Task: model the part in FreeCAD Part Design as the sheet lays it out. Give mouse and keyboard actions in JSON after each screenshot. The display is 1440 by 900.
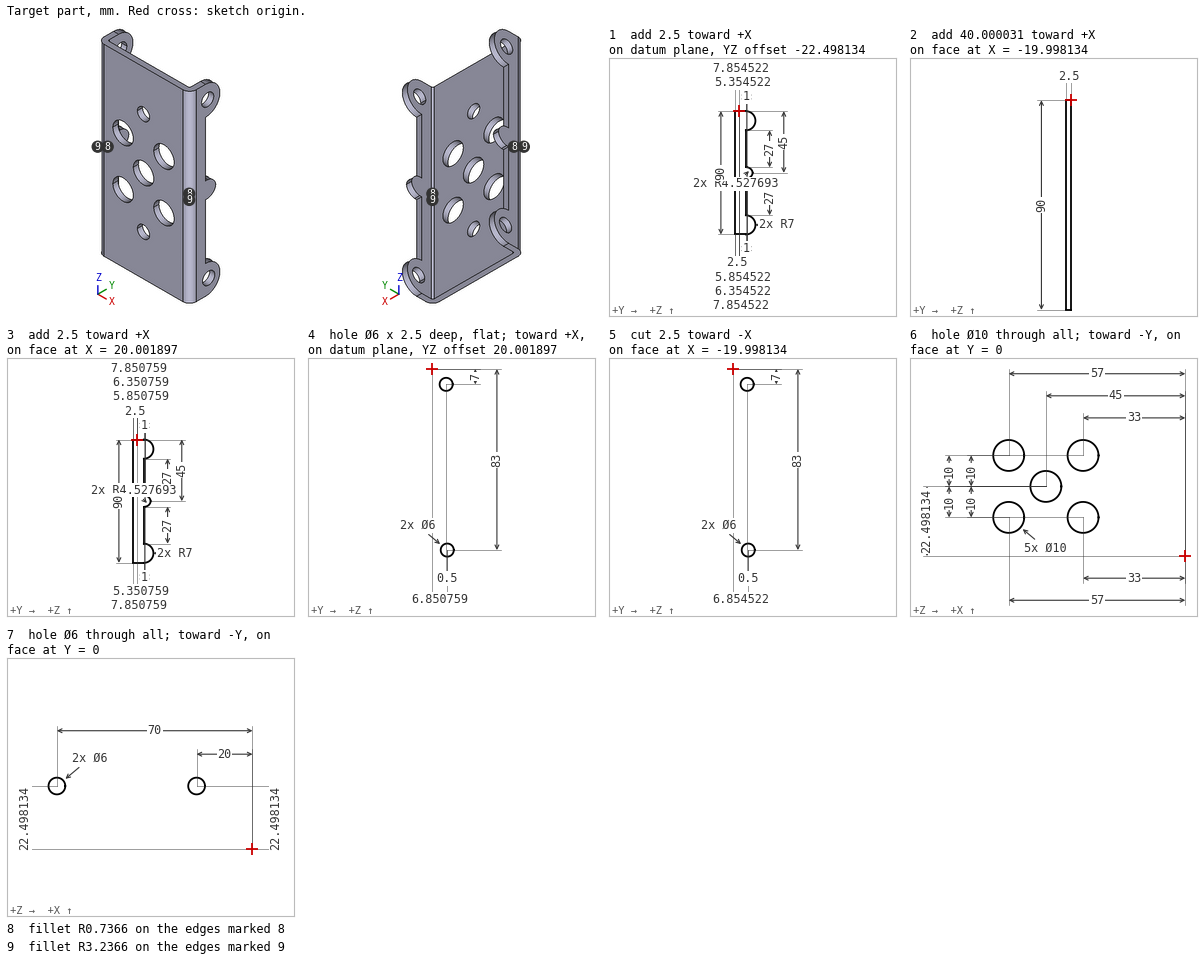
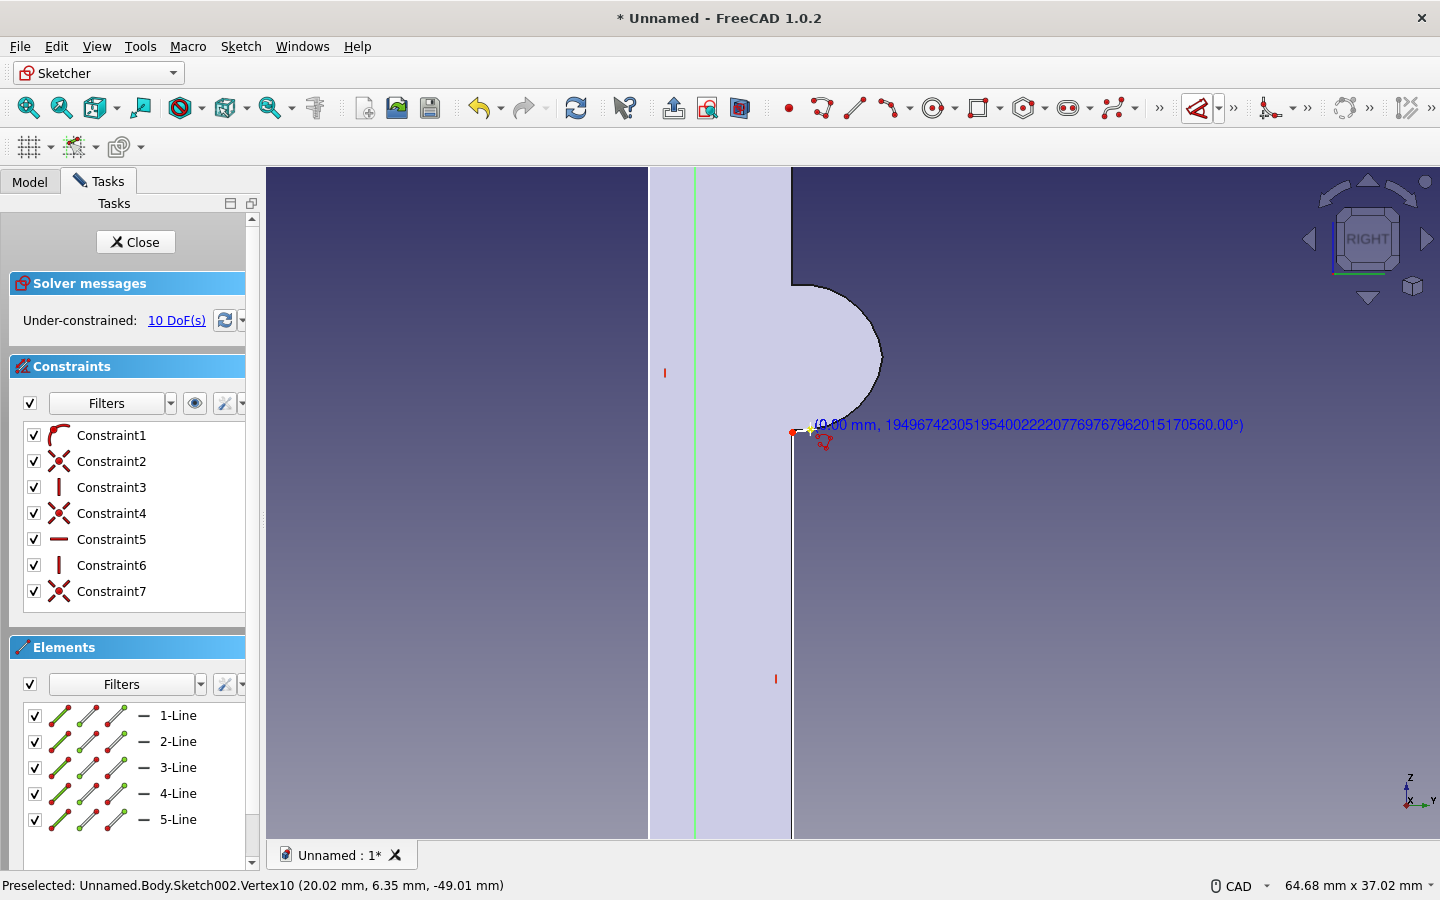
{"action": "scroll", "coordinate": [785, 551], "scroll_direction": "down", "scroll_amount": 7}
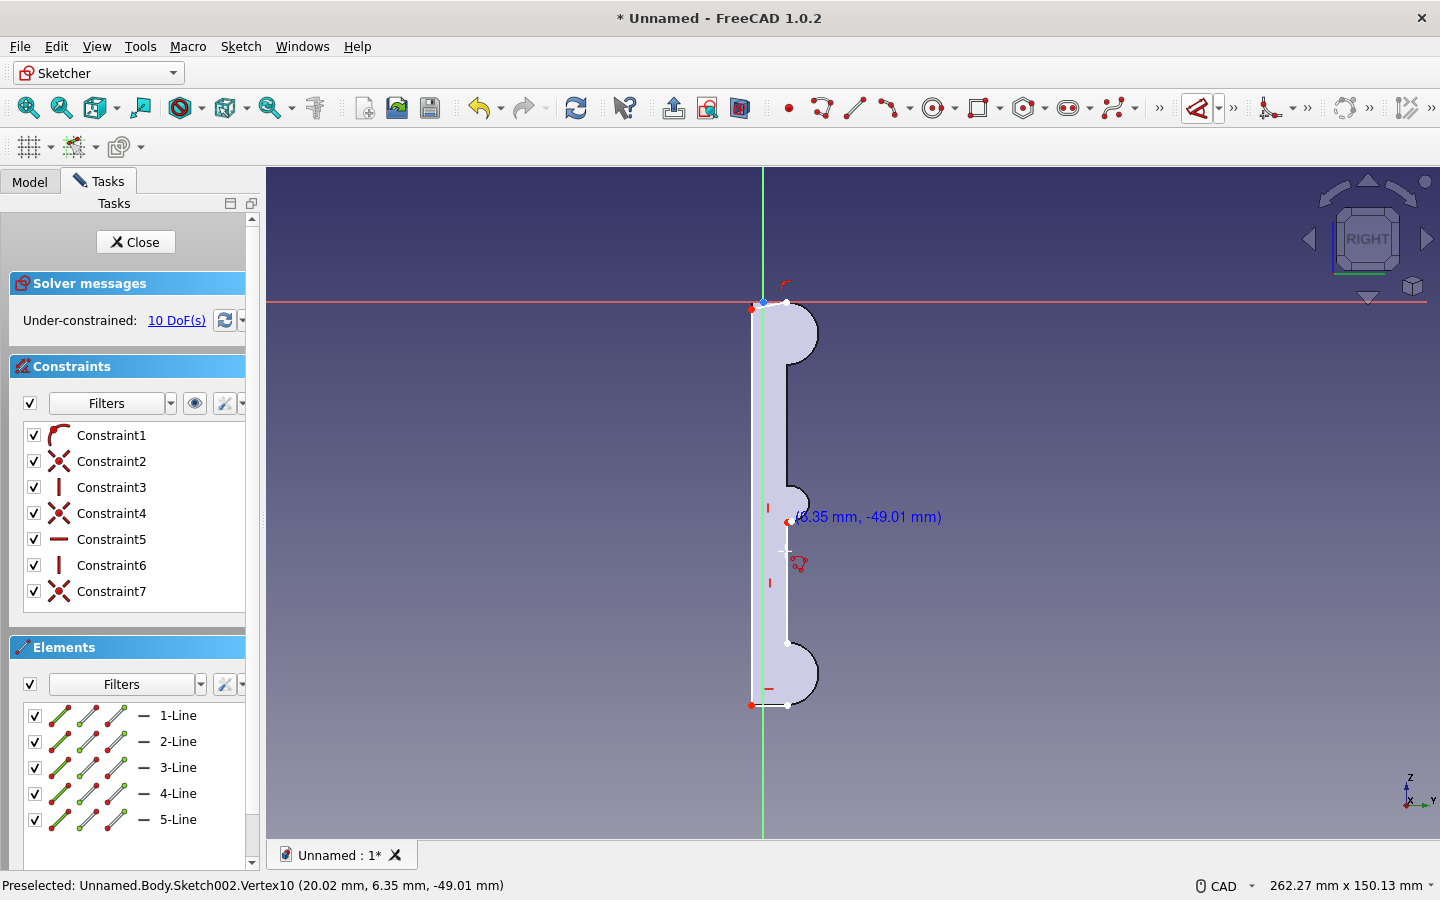
{"action": "left_click", "coordinate": [792, 486]}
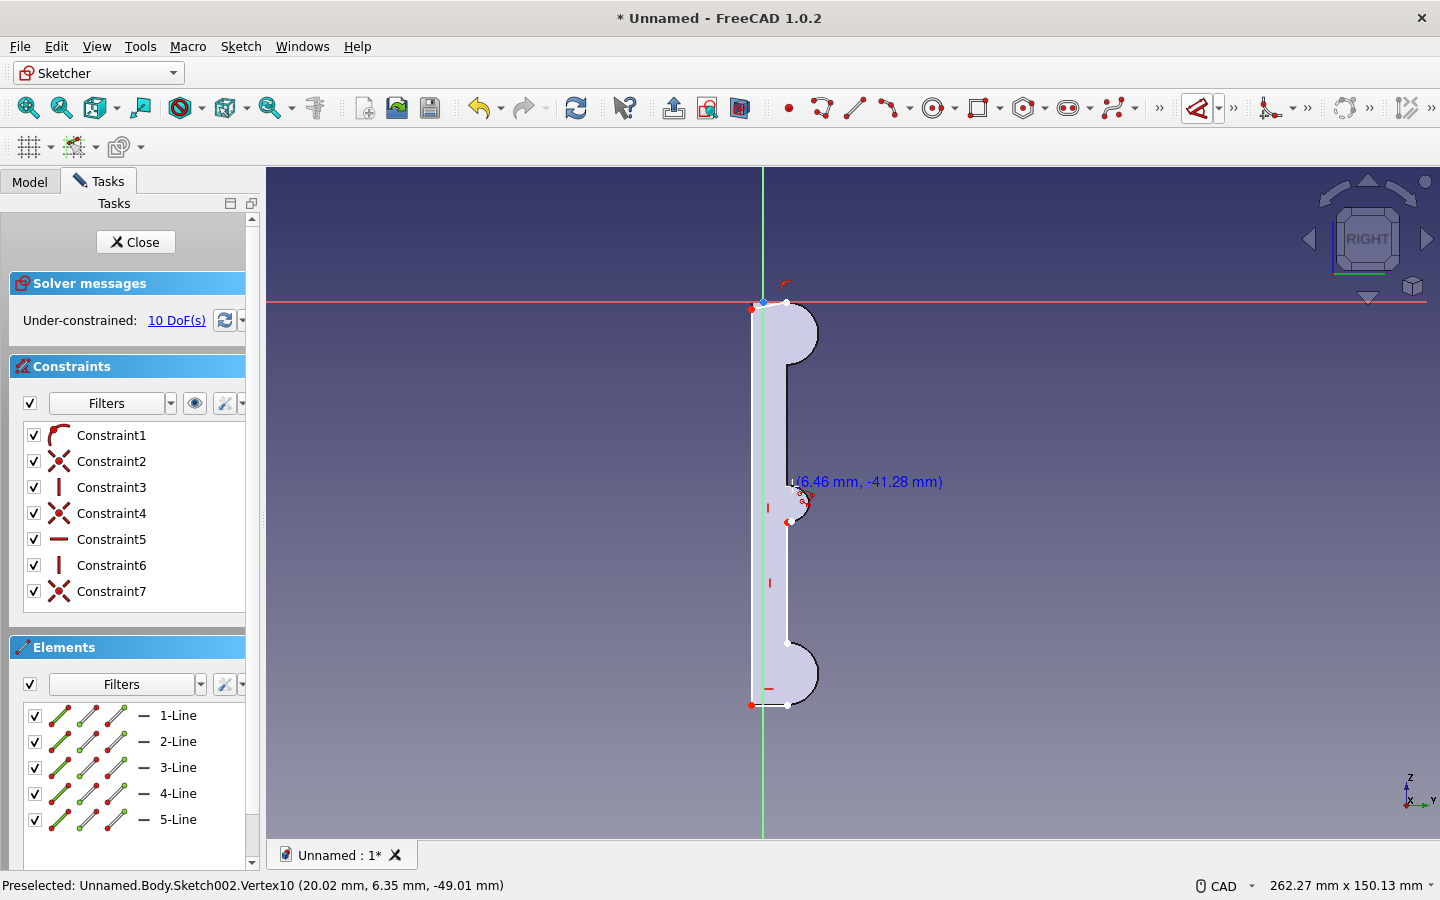
{"action": "scroll", "coordinate": [787, 486], "scroll_direction": "up", "scroll_amount": 7}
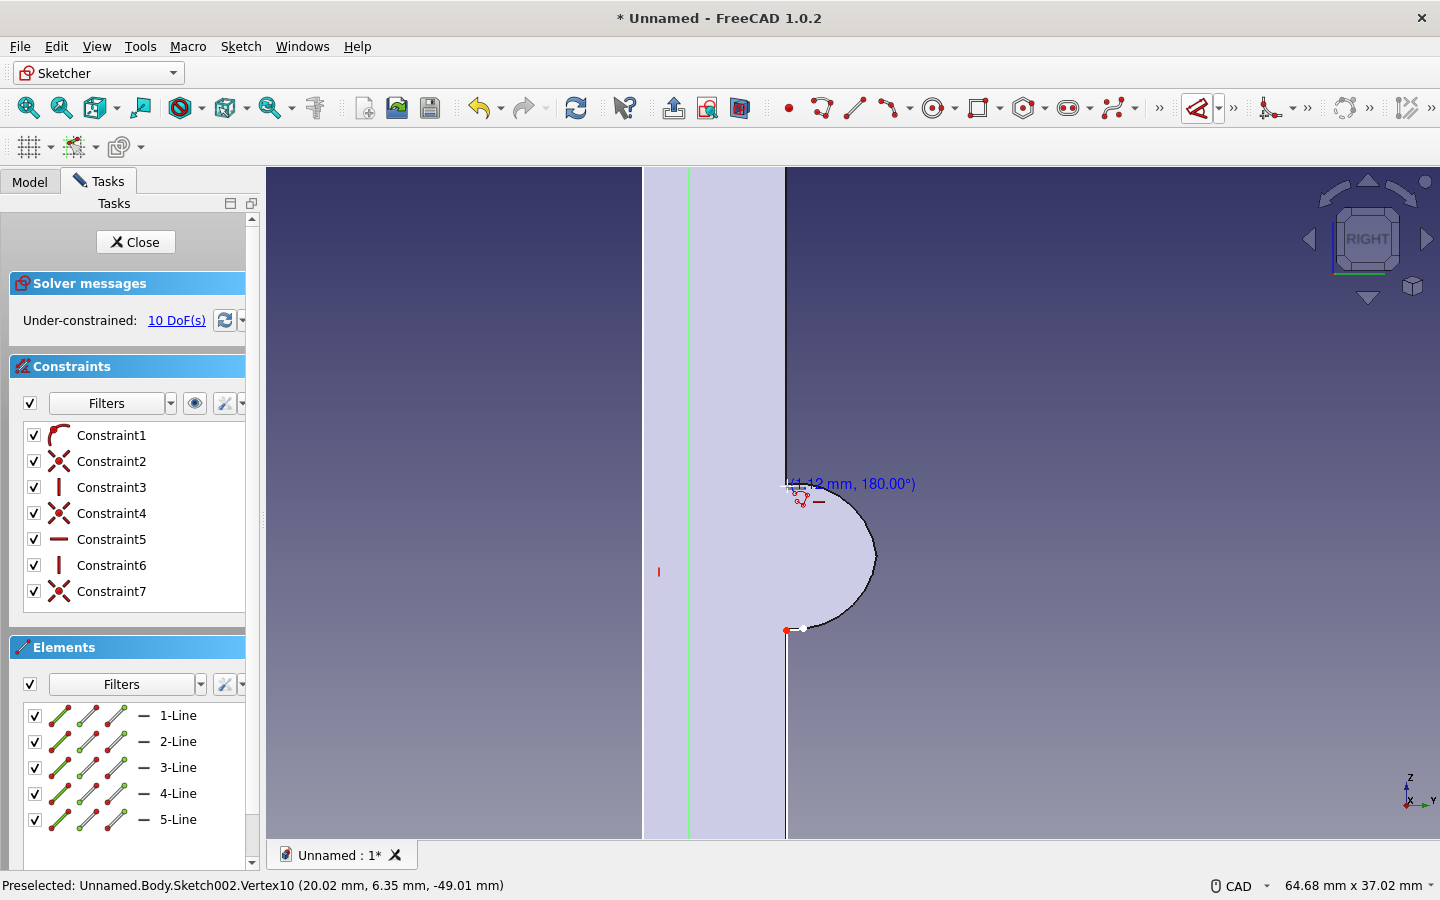
{"action": "left_click", "coordinate": [786, 485]}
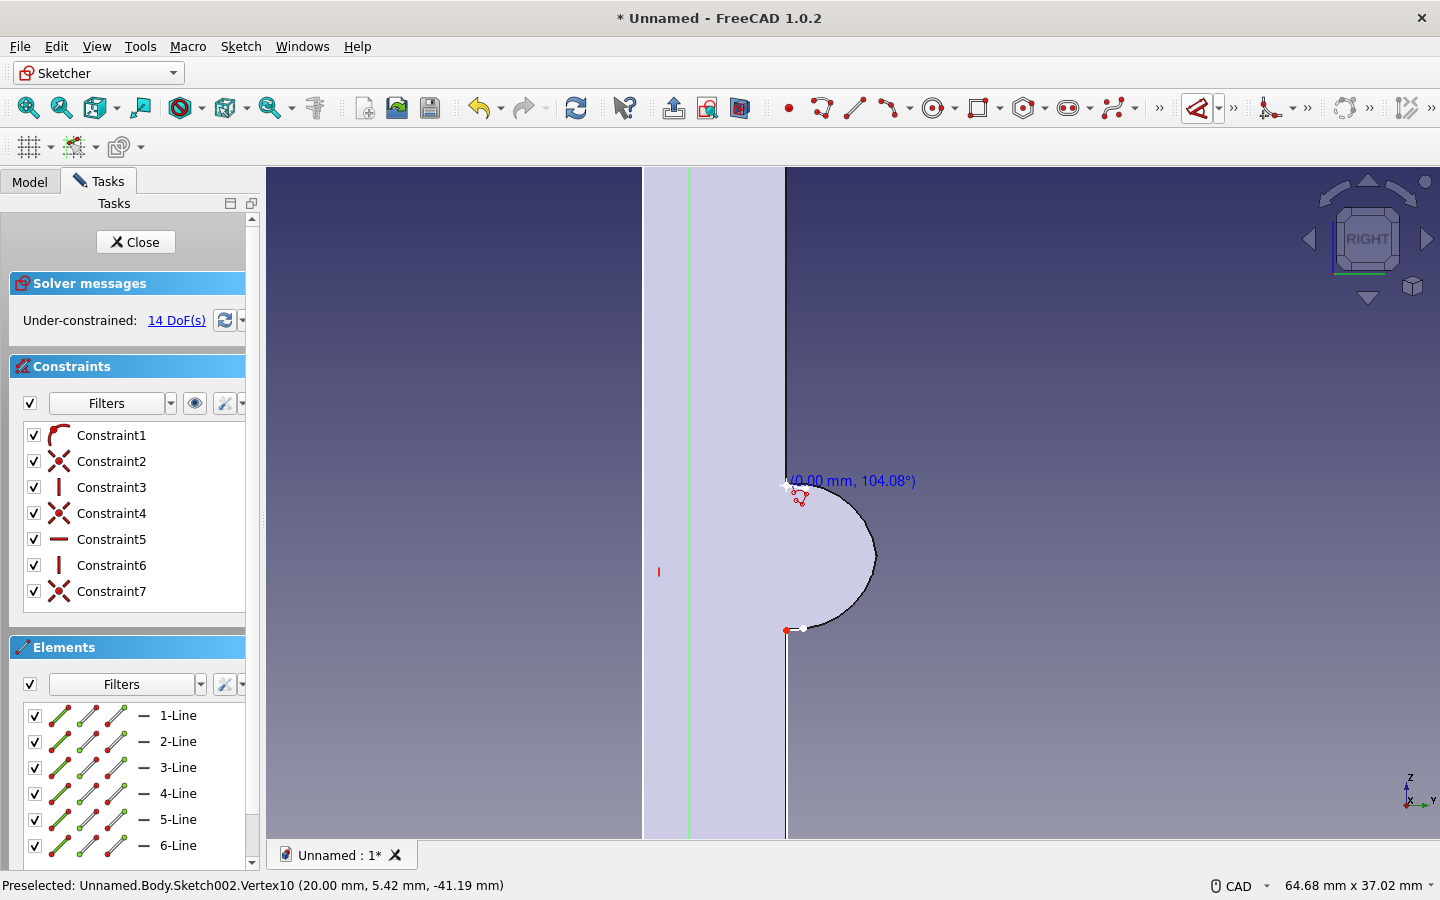
{"action": "scroll", "coordinate": [787, 486], "scroll_direction": "down", "scroll_amount": 7}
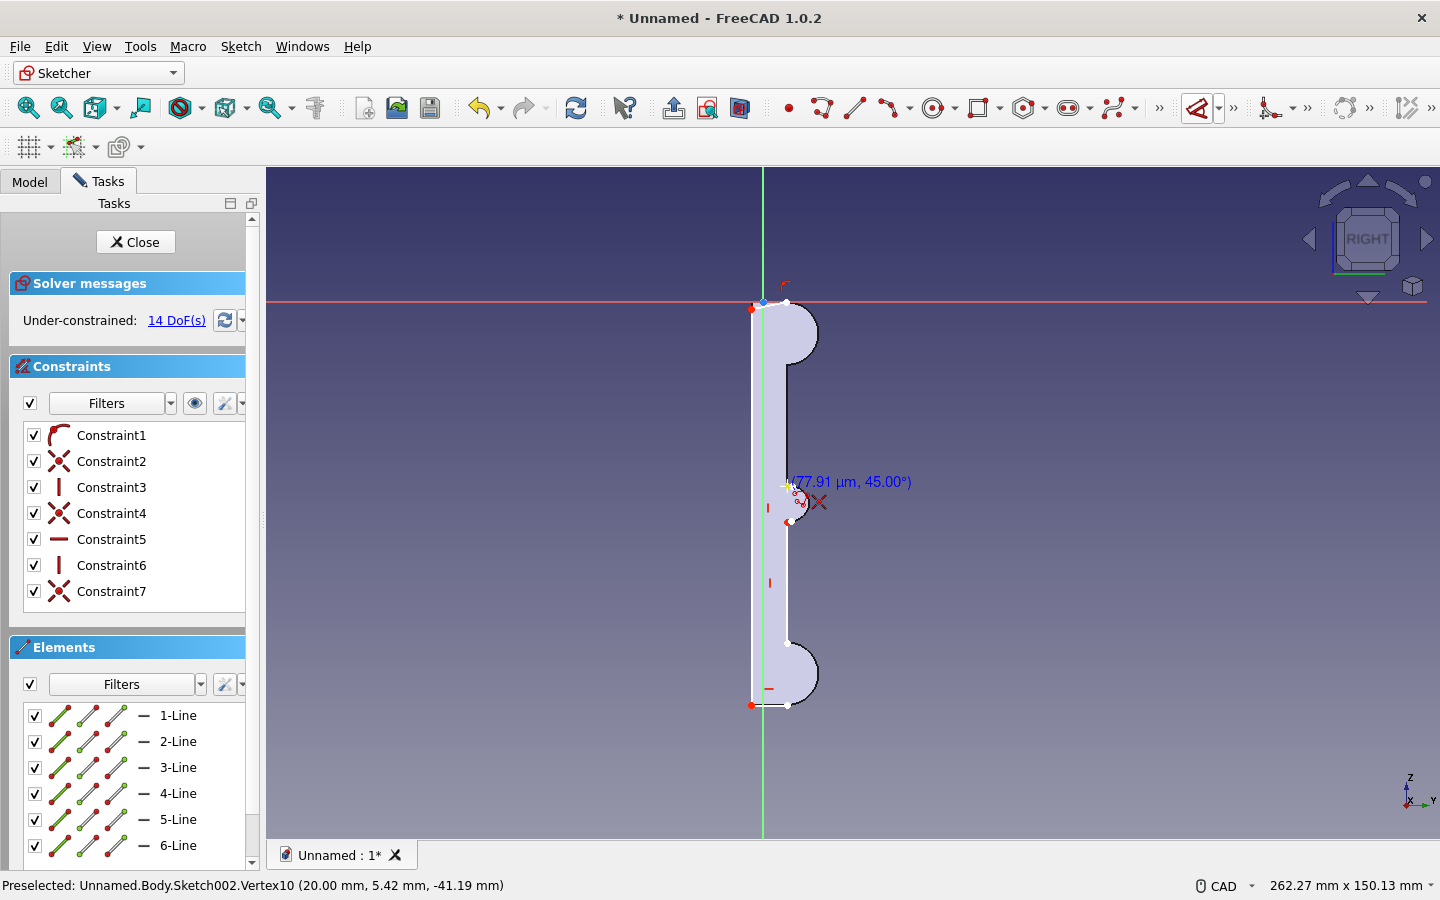
{"action": "left_click", "coordinate": [787, 365]}
{"action": "right_click", "coordinate": [787, 365]}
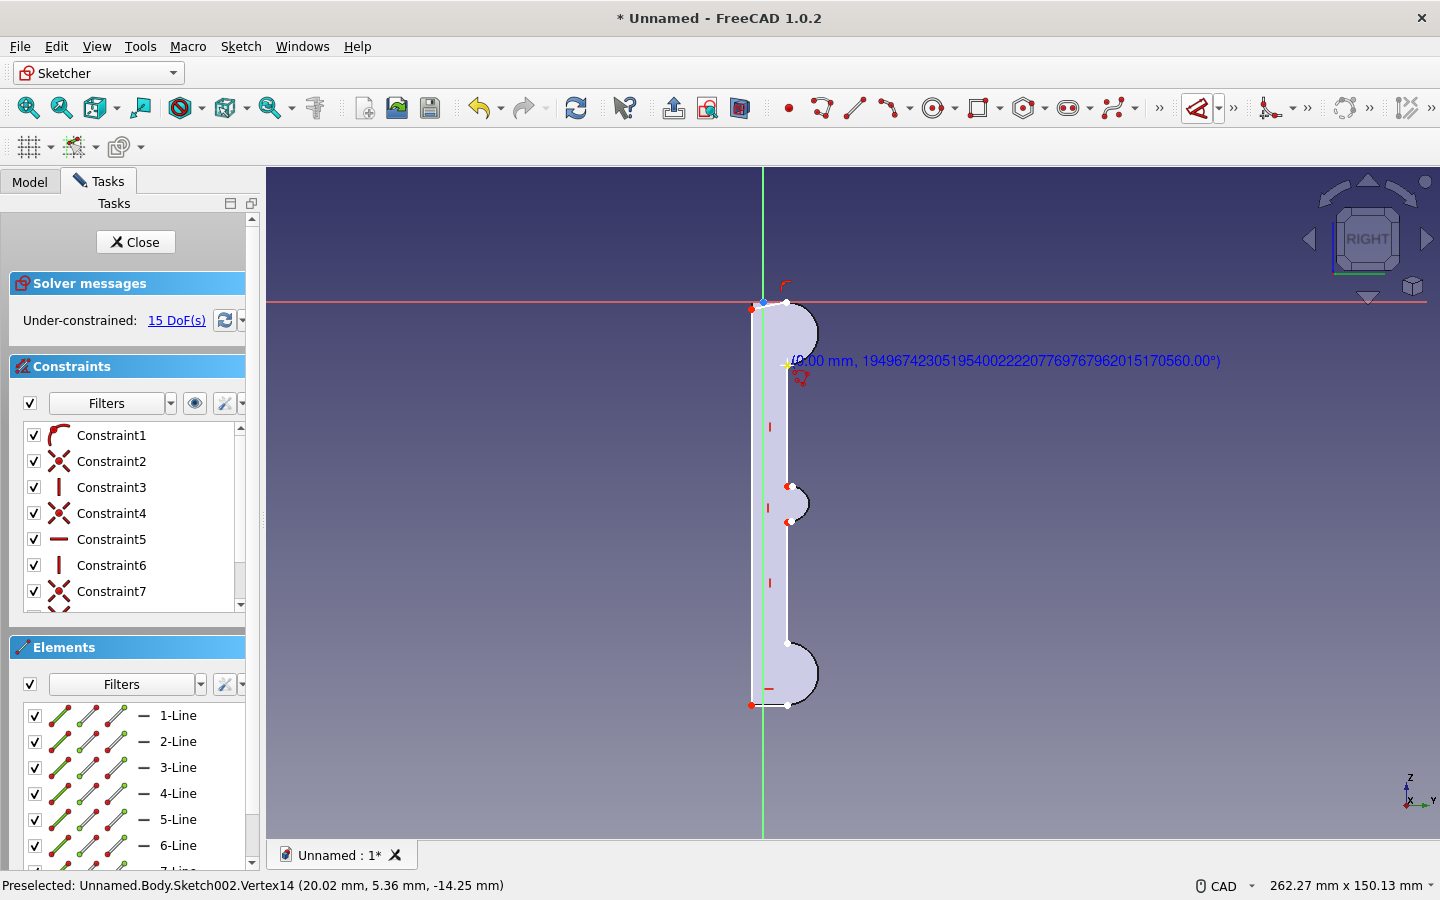
{"action": "key", "text": "g 3 a"}